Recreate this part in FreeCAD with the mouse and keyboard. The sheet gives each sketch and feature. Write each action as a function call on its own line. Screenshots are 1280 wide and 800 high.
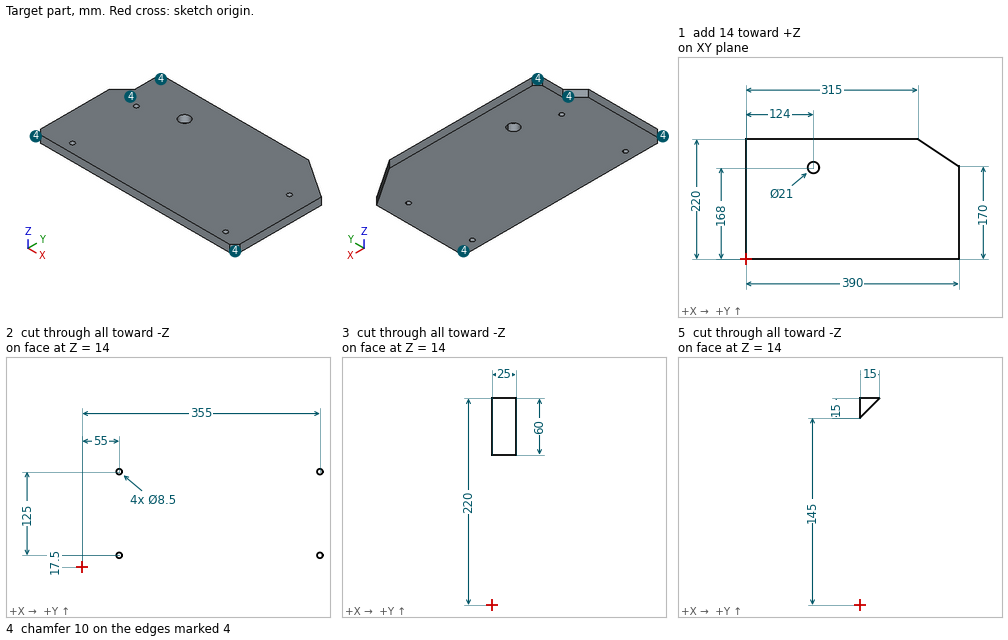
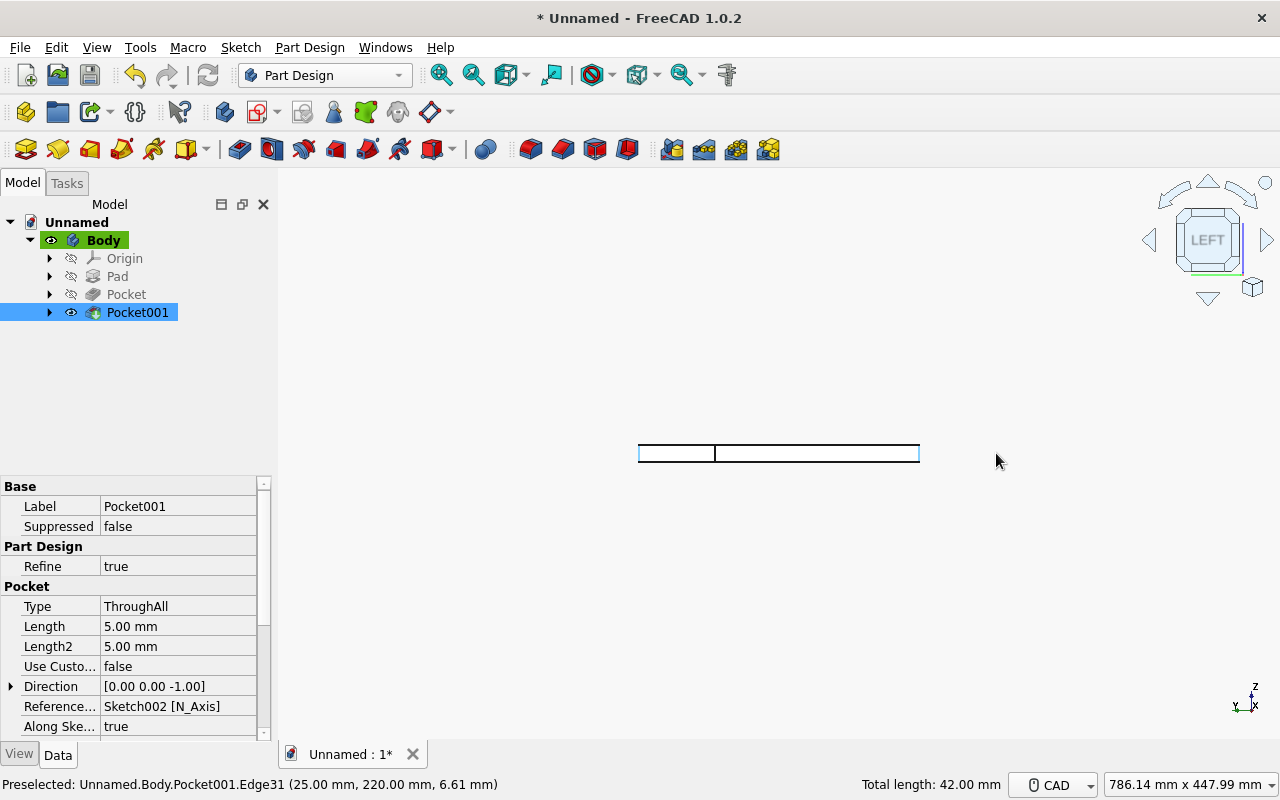
key(v)
key(f)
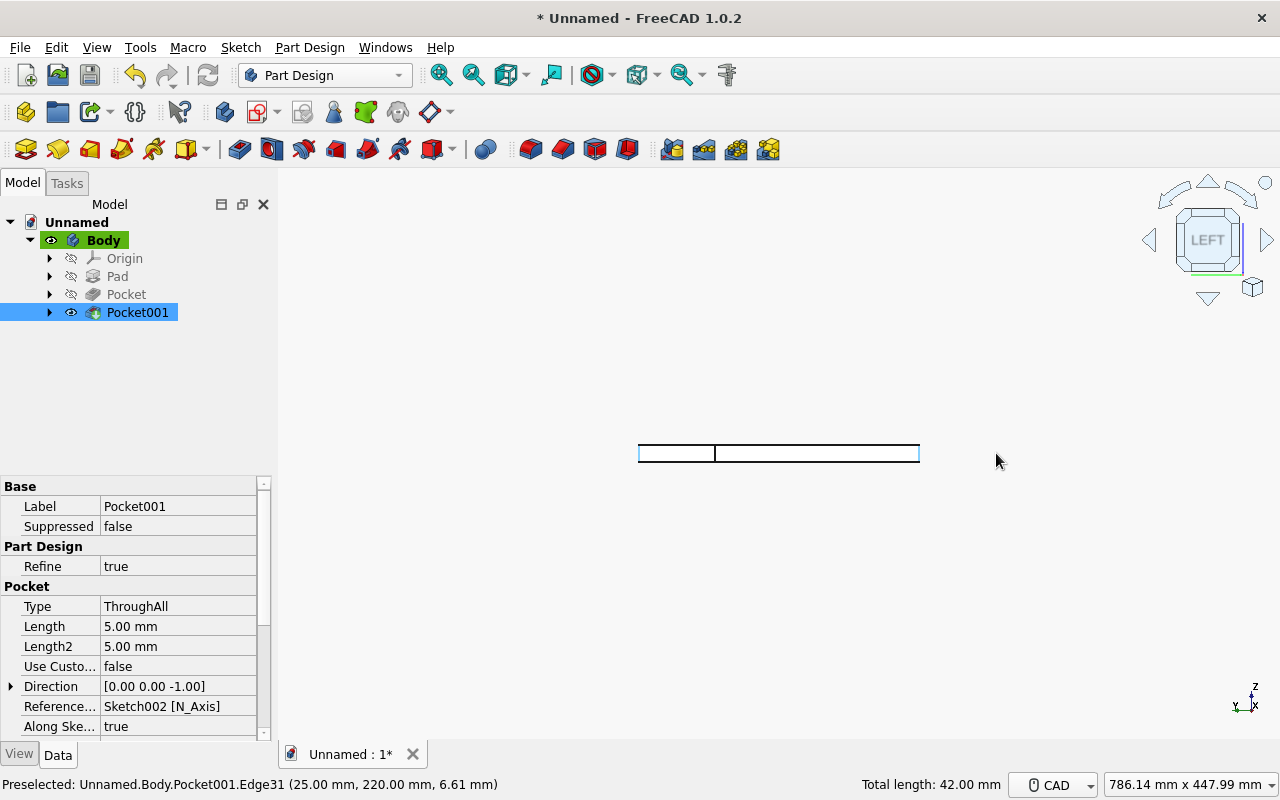
scroll(715, 452, up, 5)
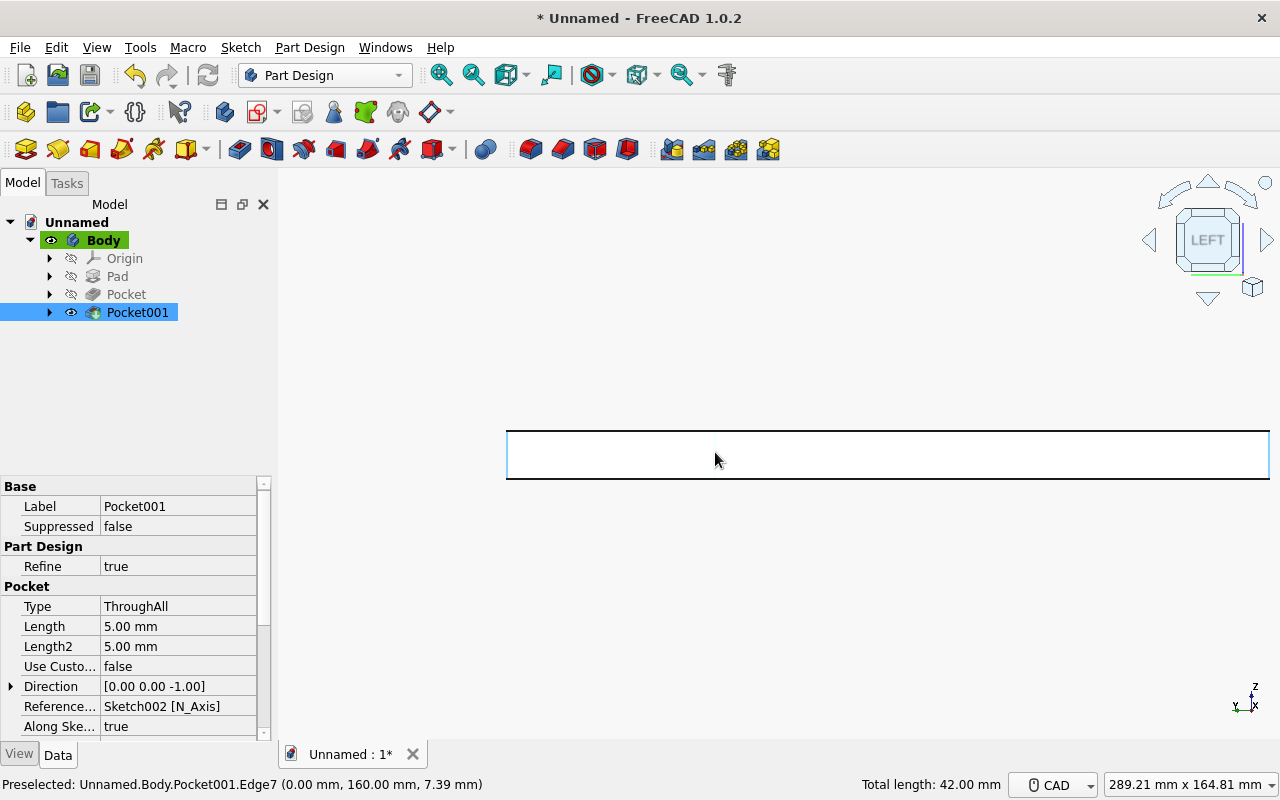
key(v)
key(f)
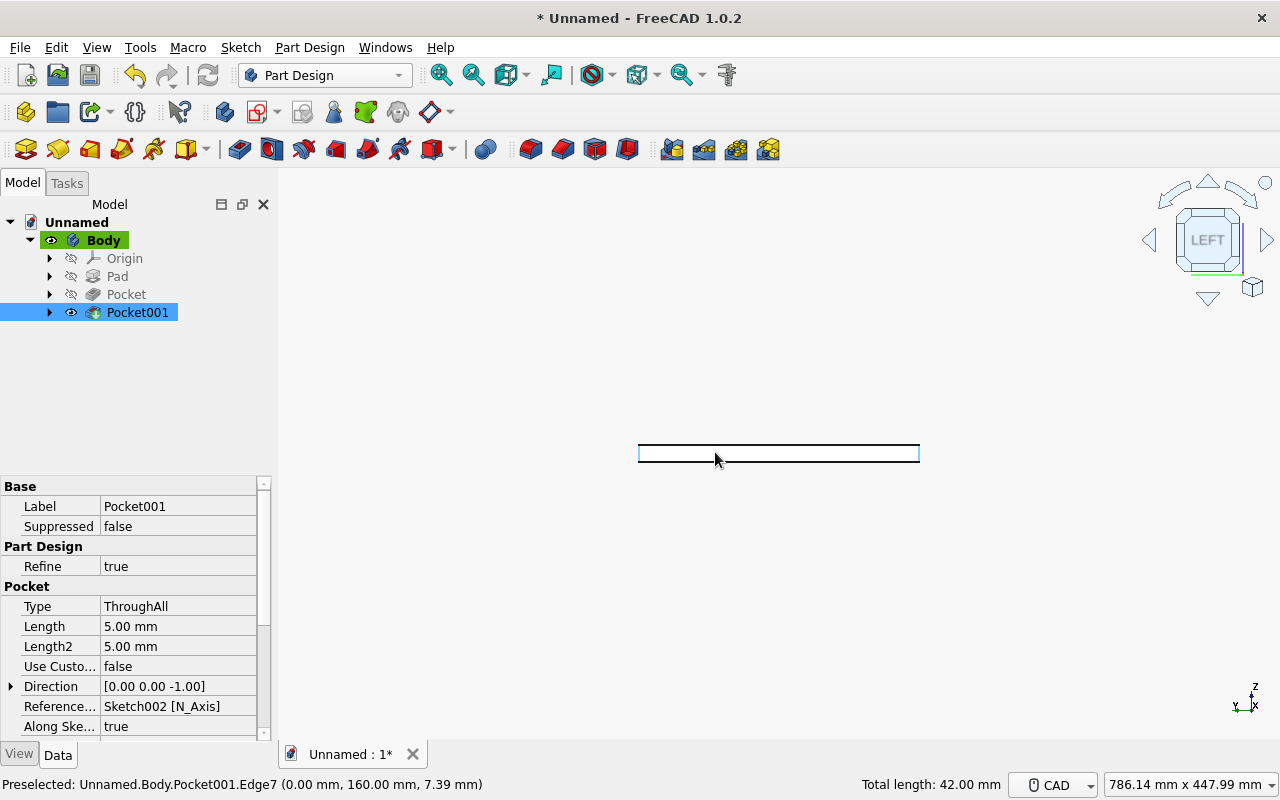
key(v)
key(3)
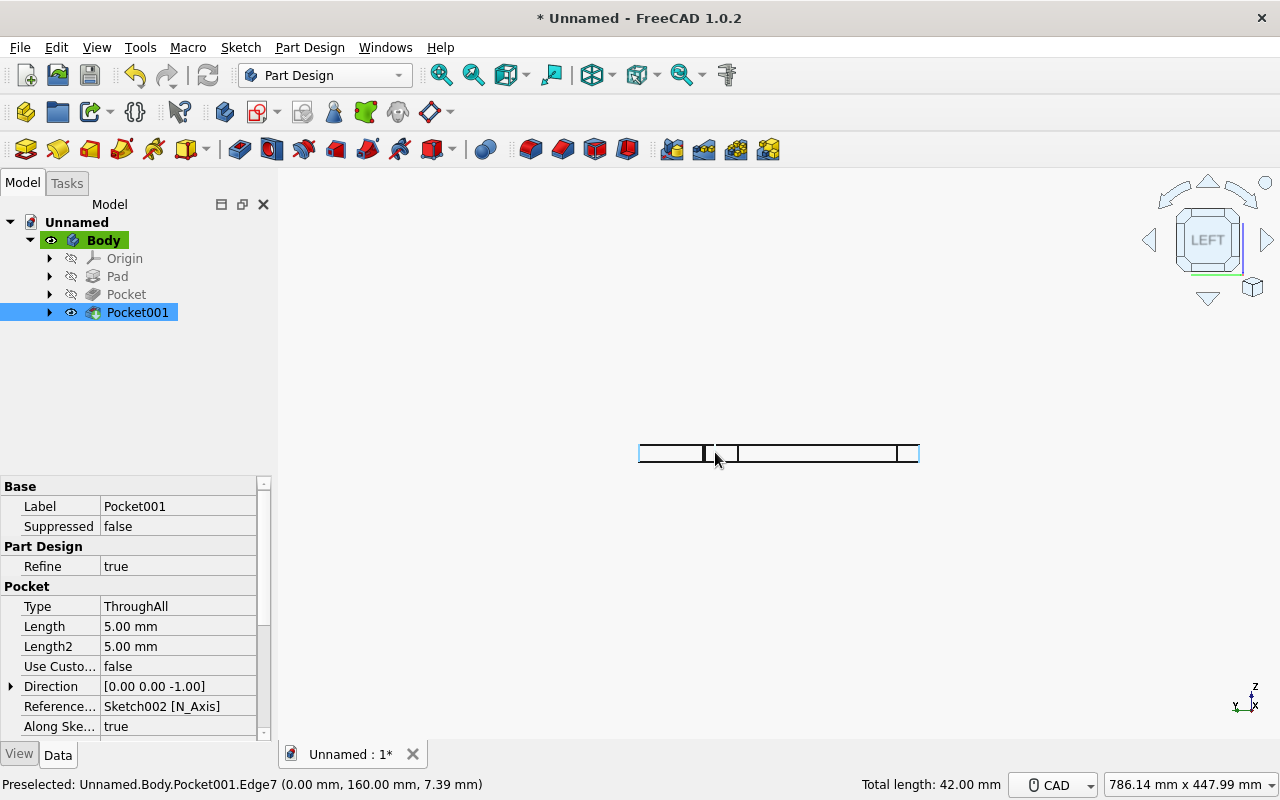
key(0)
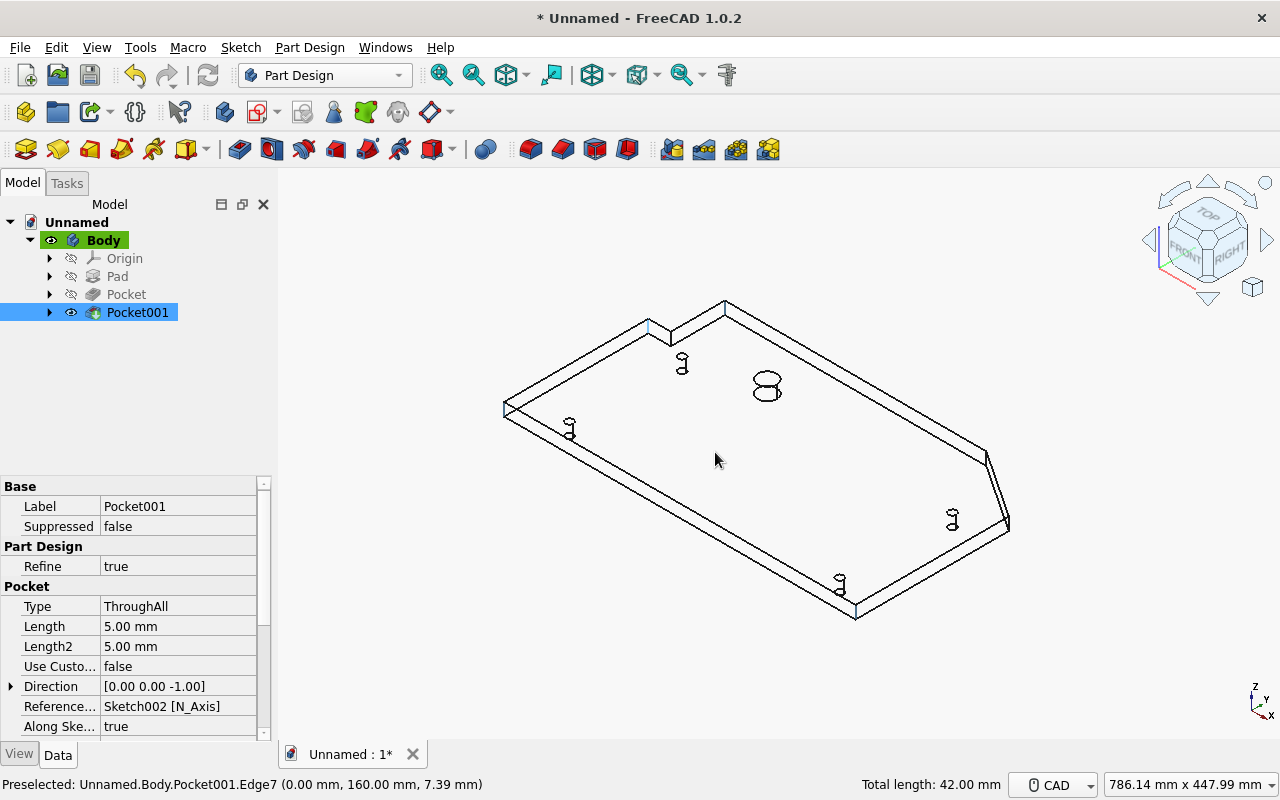
click(671, 338, ctrl)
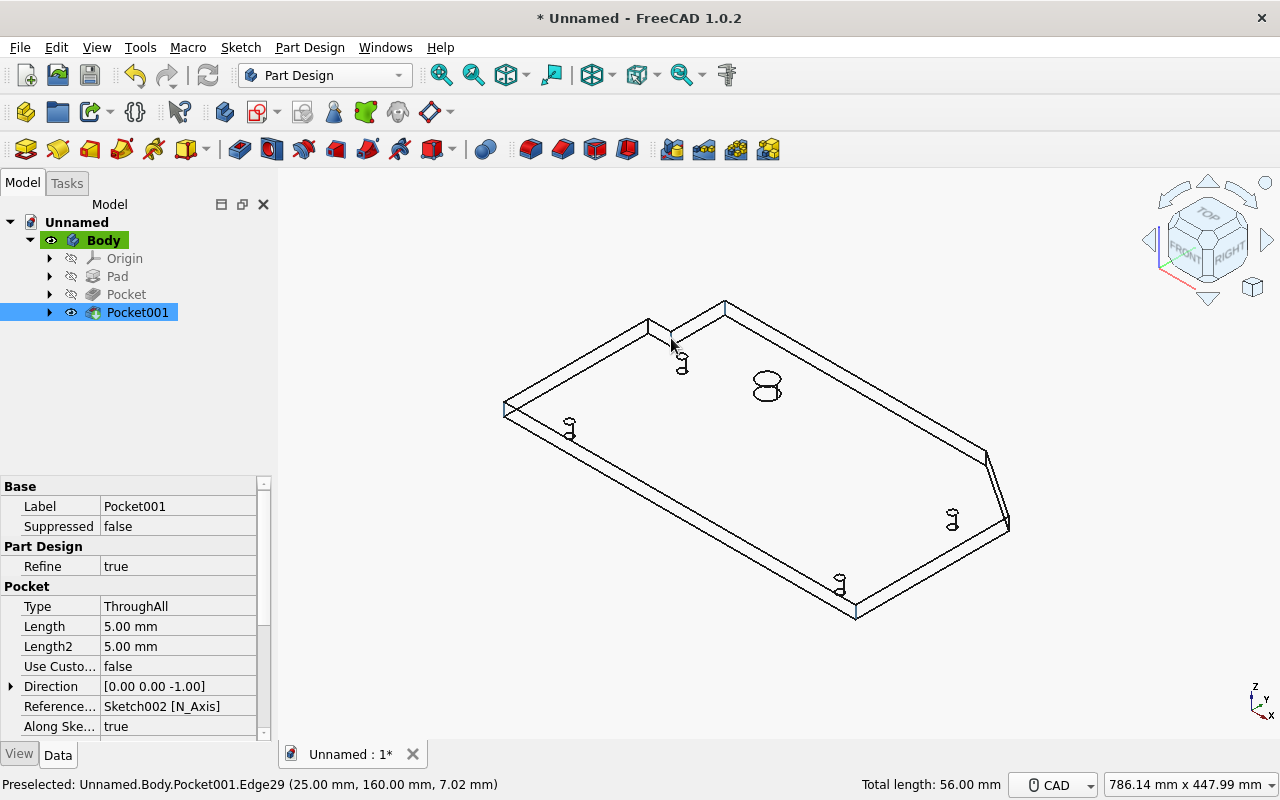
key(v)
key(1)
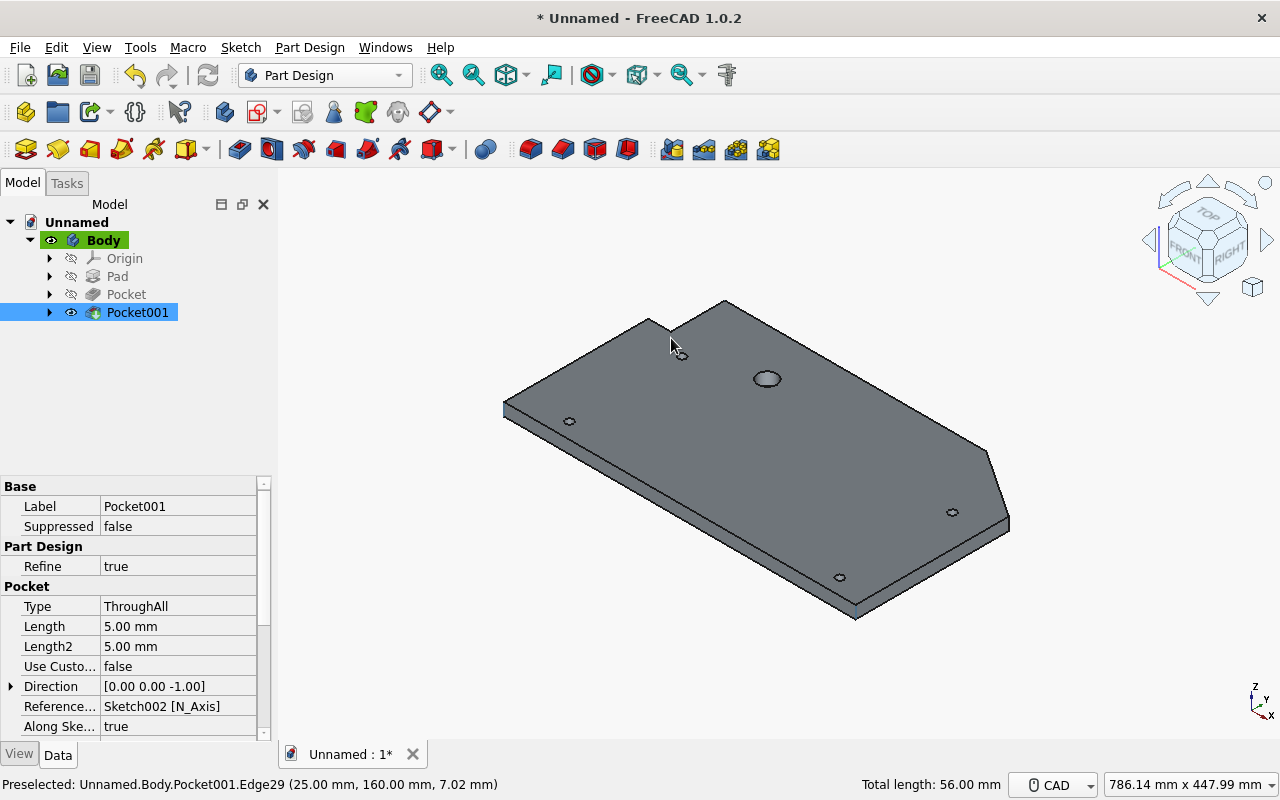
click(564, 150)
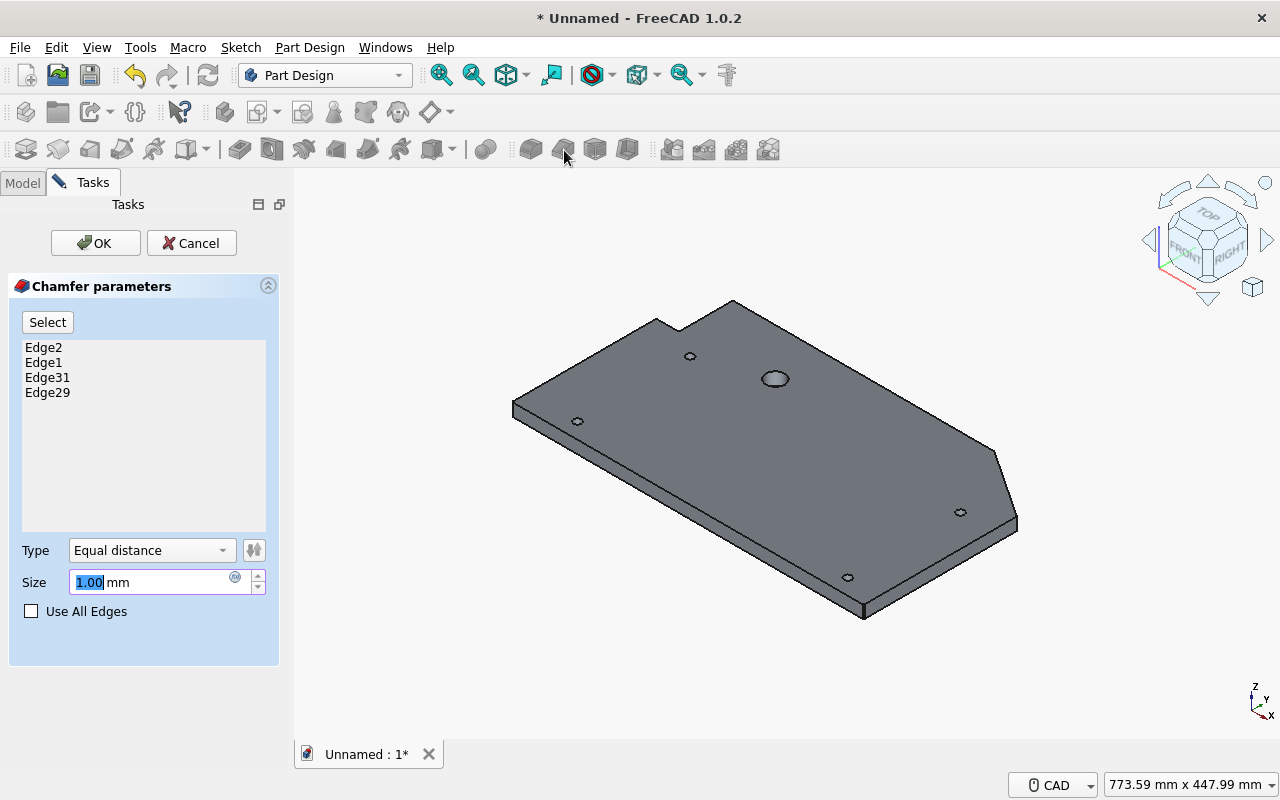
text(10)
key(Tab)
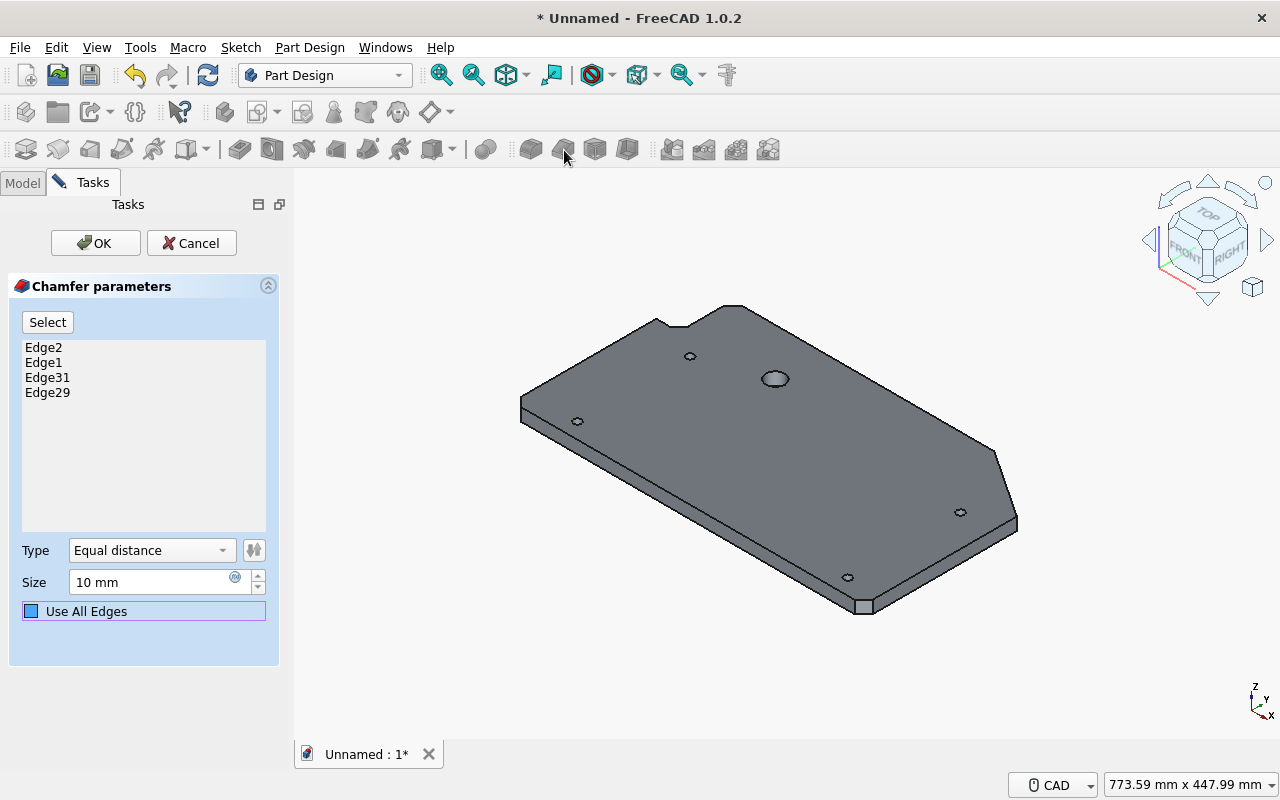
click(96, 243)